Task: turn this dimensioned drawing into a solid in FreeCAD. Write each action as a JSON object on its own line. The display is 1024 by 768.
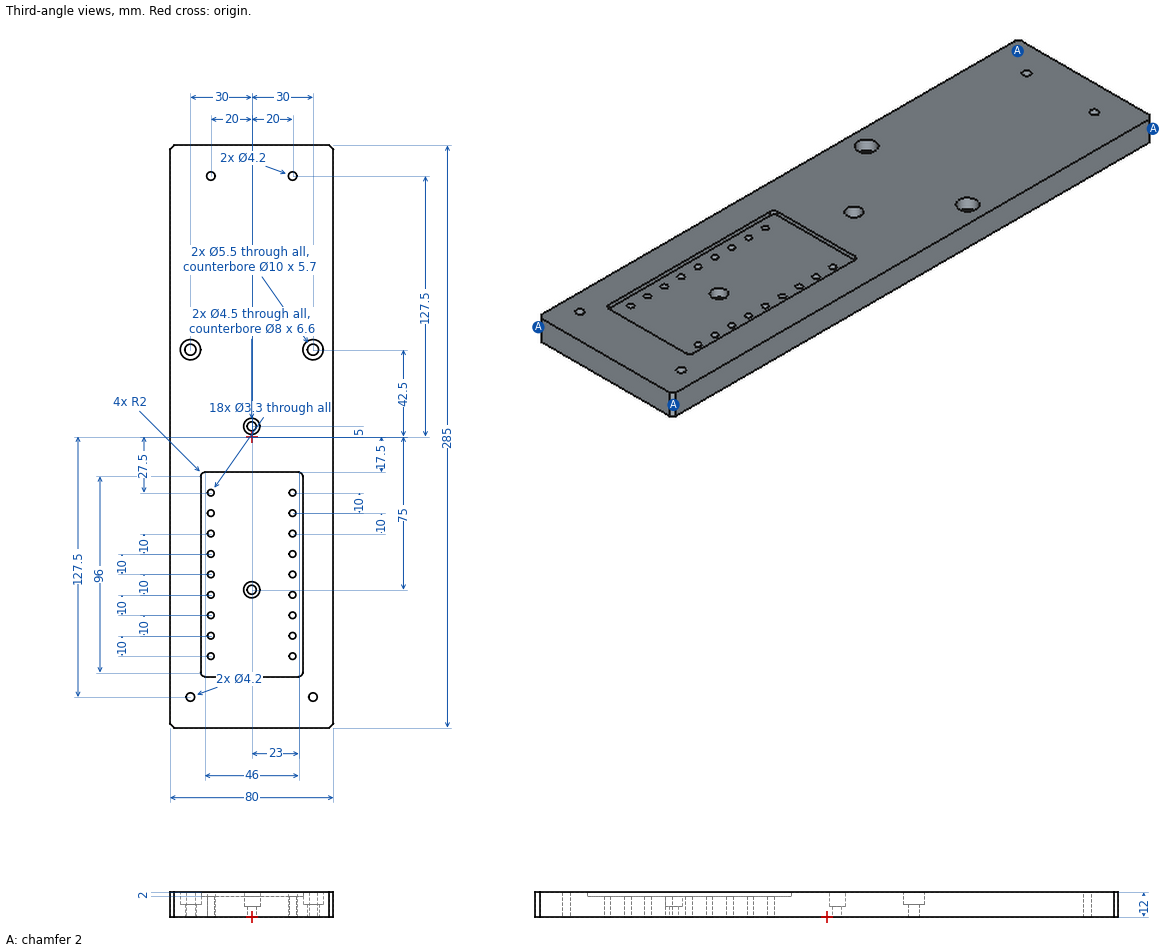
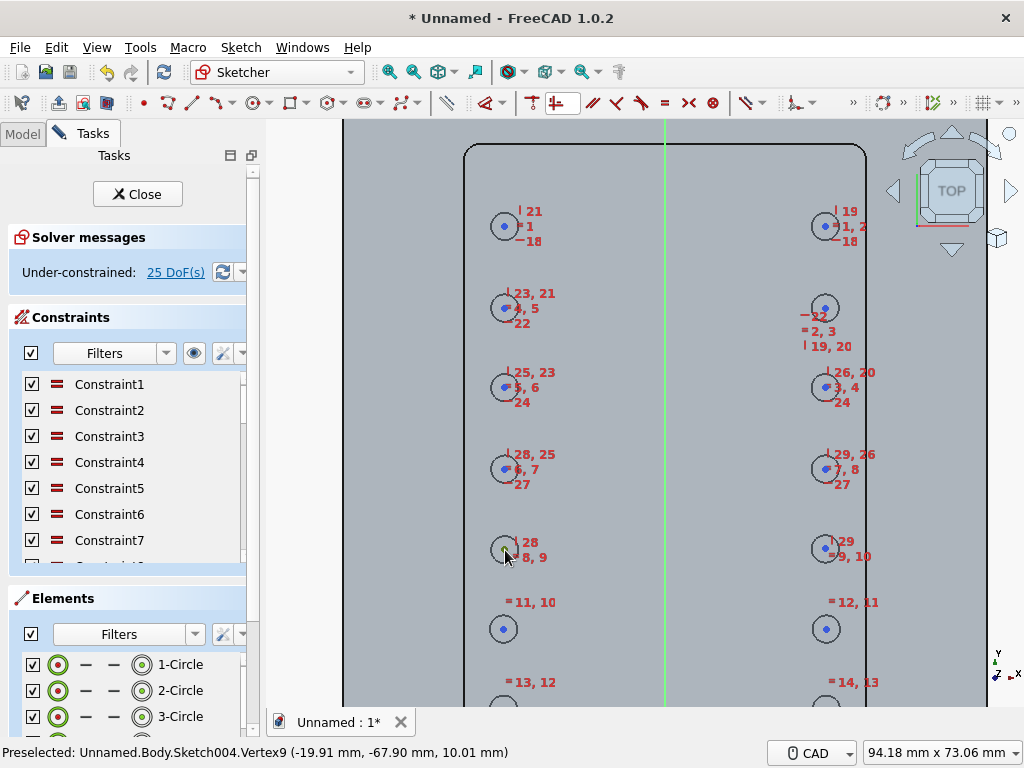
{"action": "left_click", "coordinate": [825, 549]}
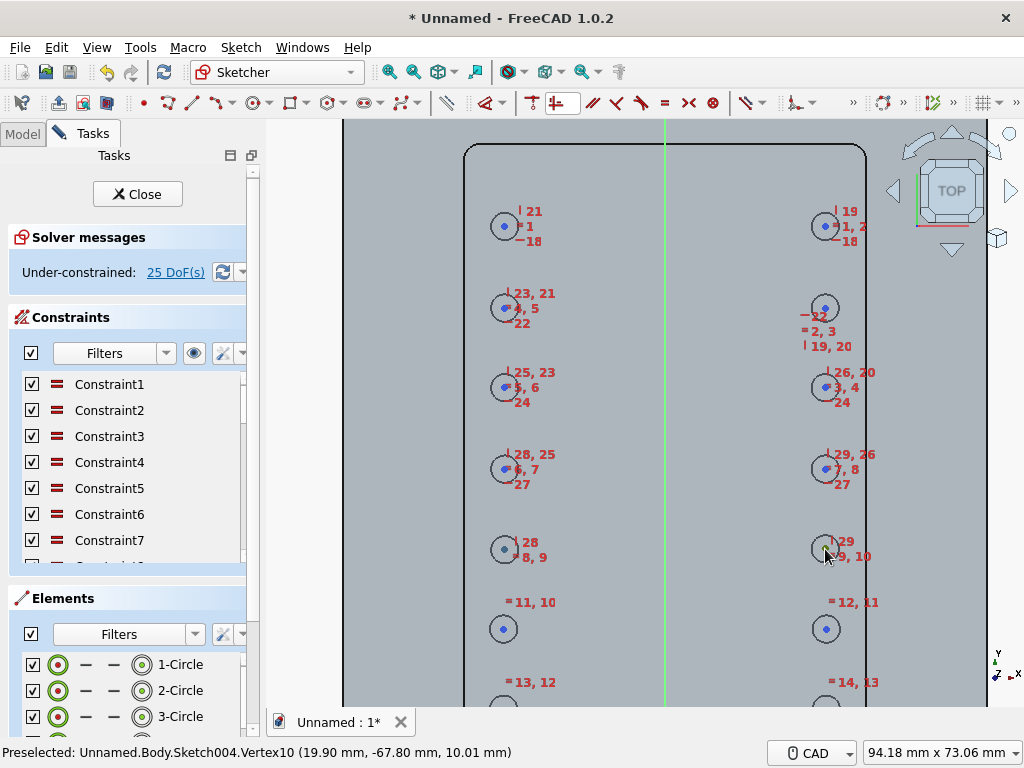
{"action": "key", "text": "h"}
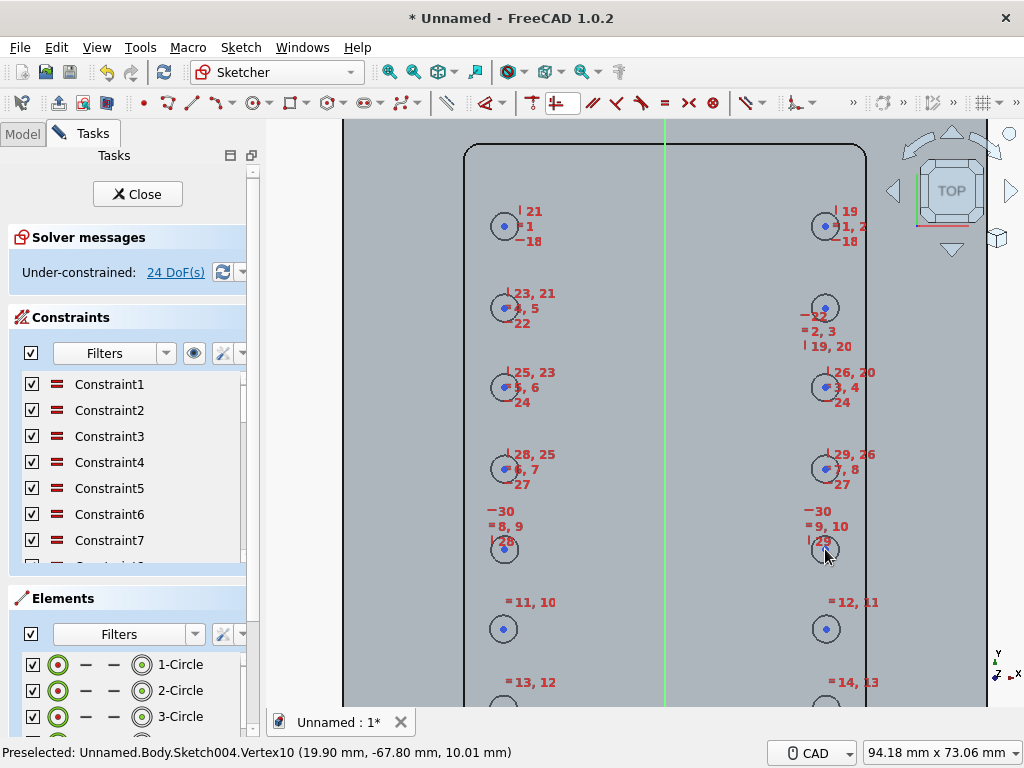
{"action": "left_click", "coordinate": [505, 550]}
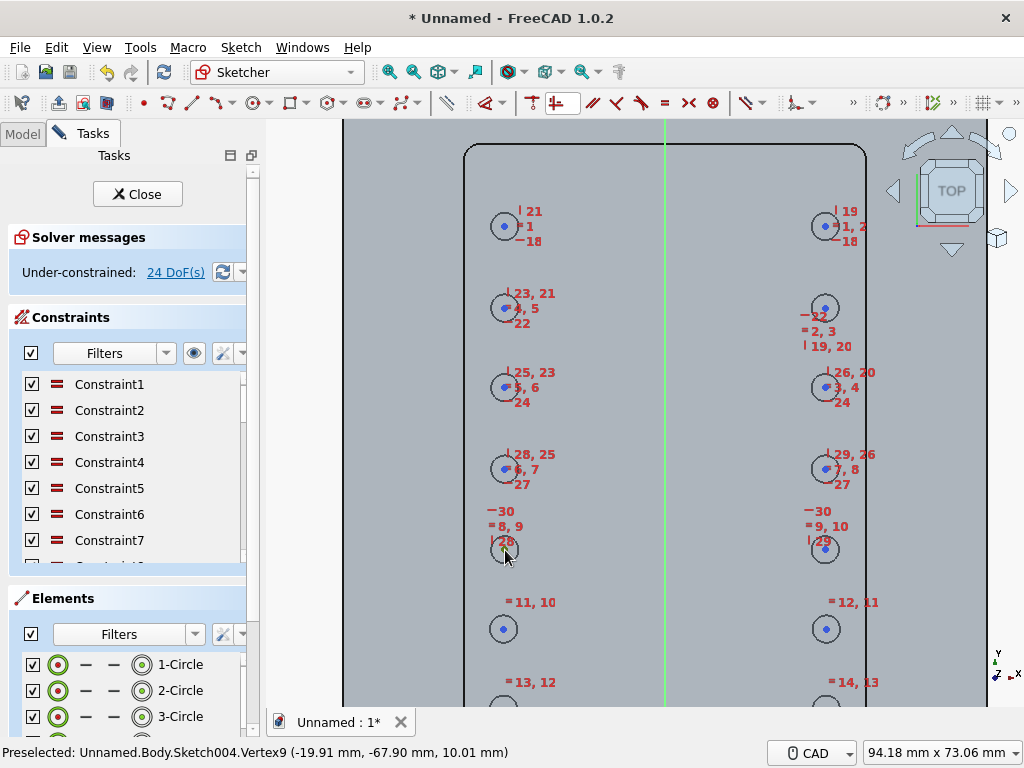
{"action": "left_click", "coordinate": [504, 629]}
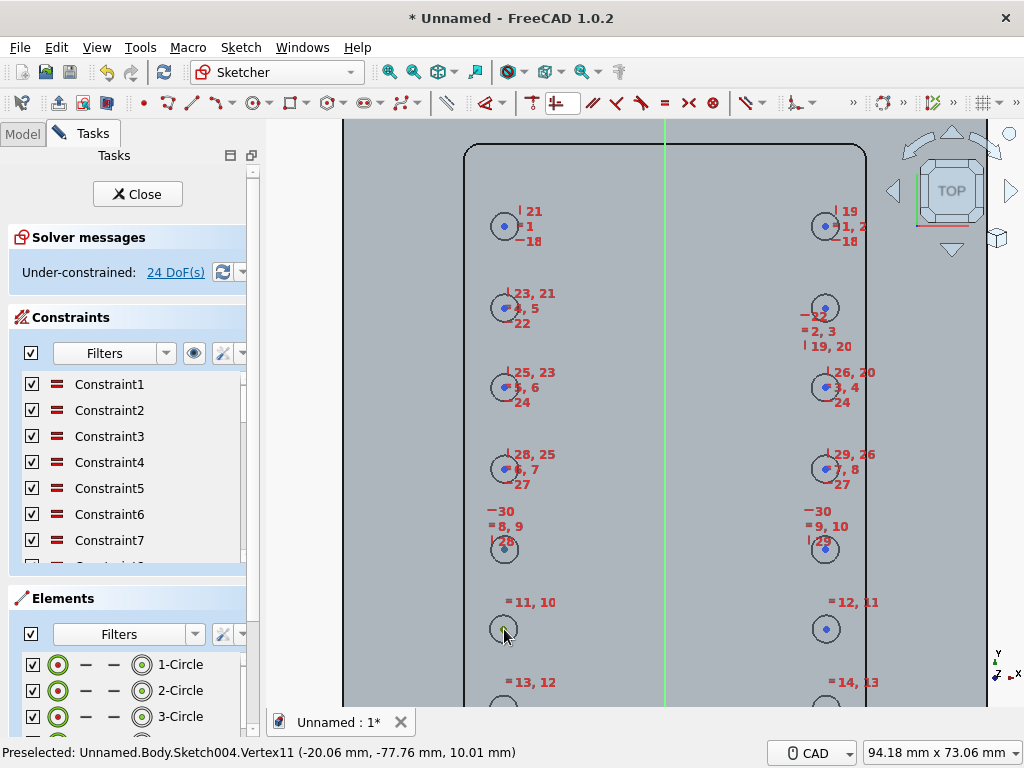
{"action": "left_click", "coordinate": [574, 104]}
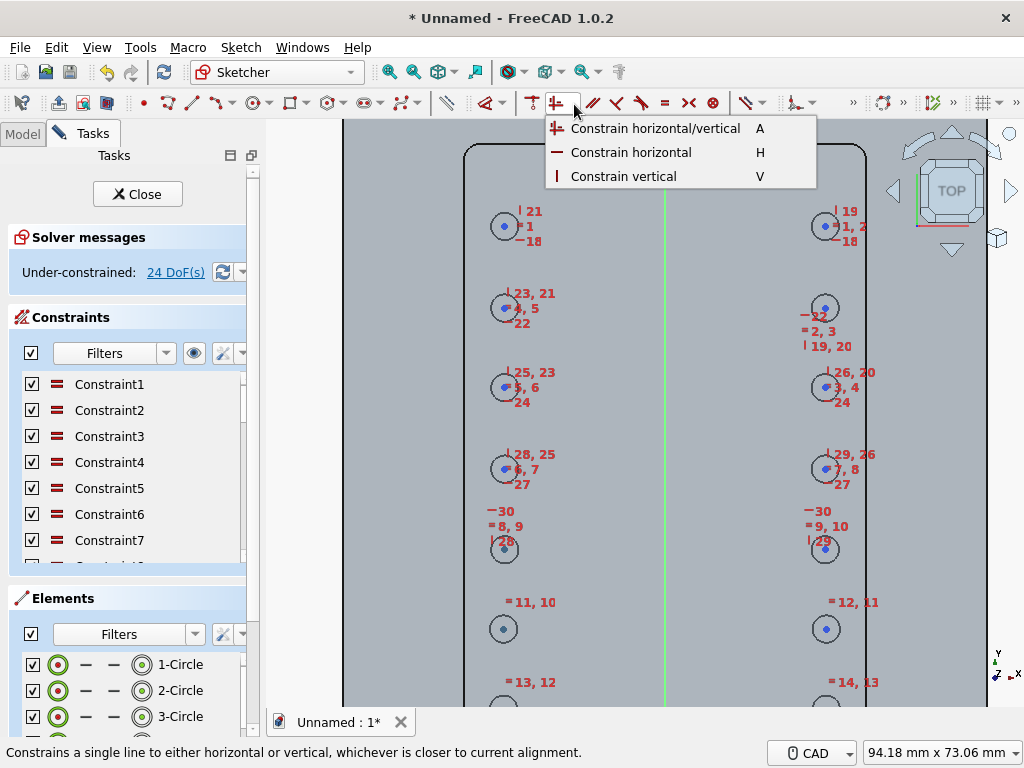
{"action": "left_click", "coordinate": [681, 176]}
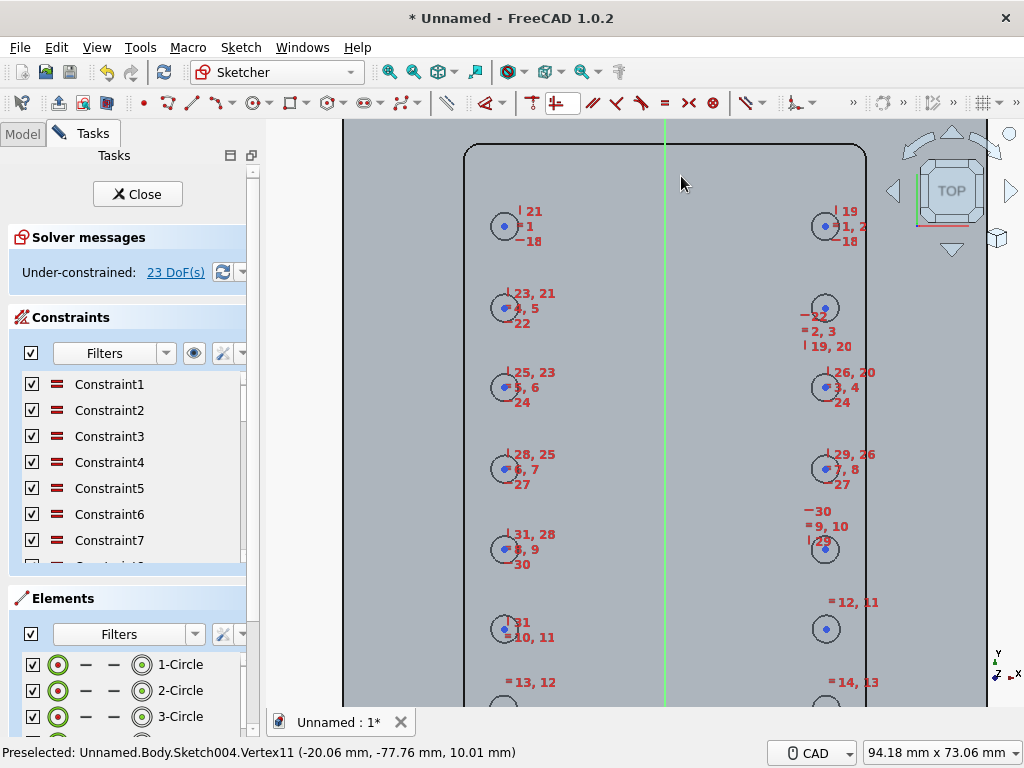
{"action": "left_click", "coordinate": [825, 550]}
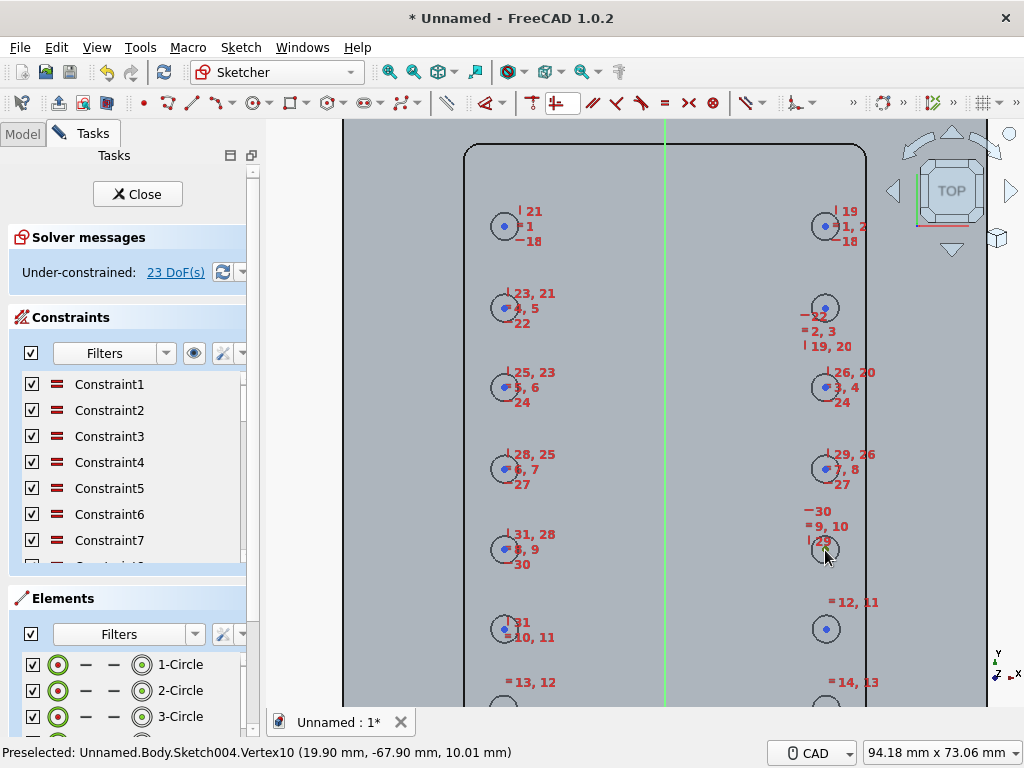
{"action": "left_click", "coordinate": [826, 629]}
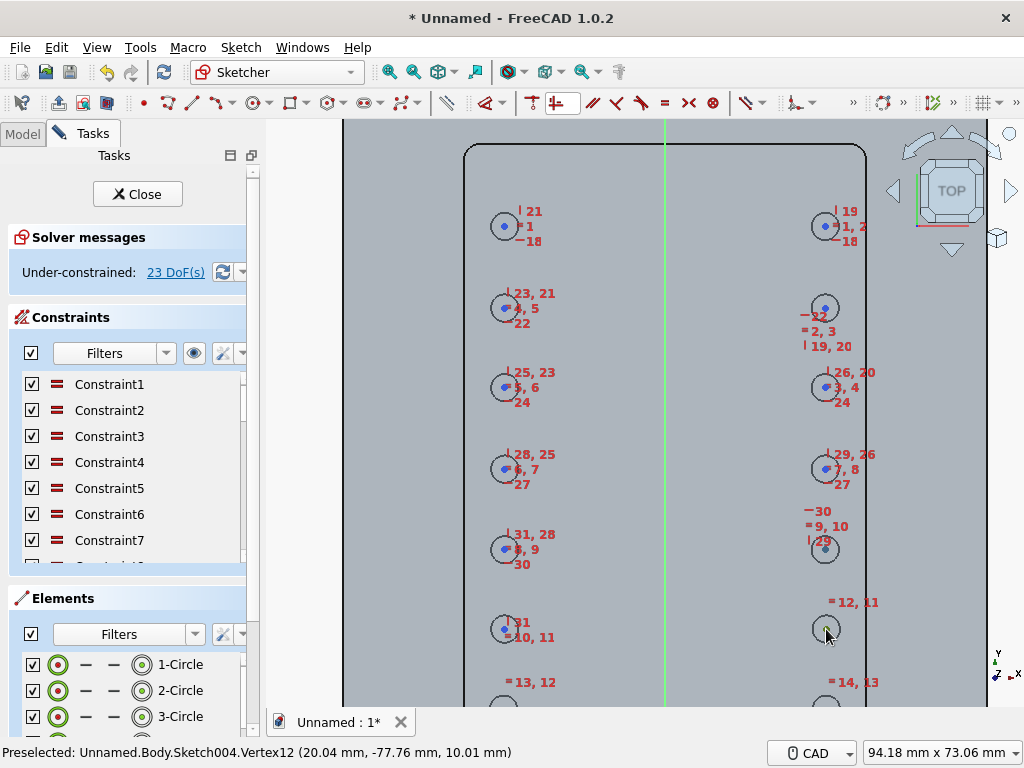
{"action": "key", "text": "v"}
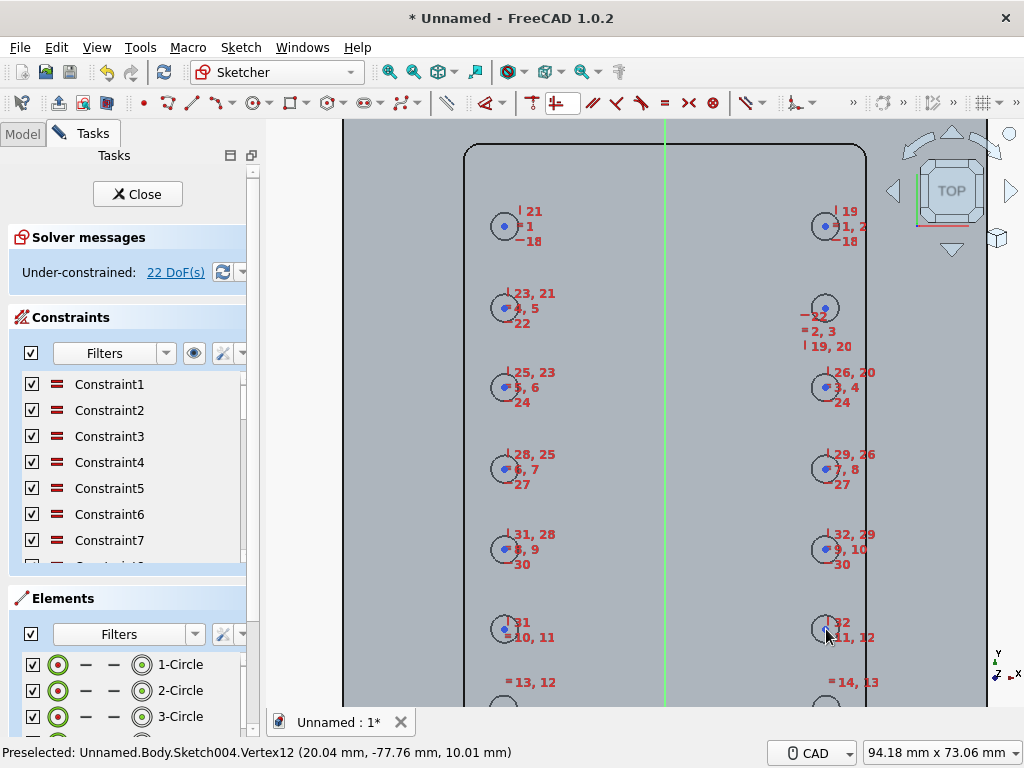
{"action": "scroll", "coordinate": [505, 629], "scroll_direction": "up", "scroll_amount": 4}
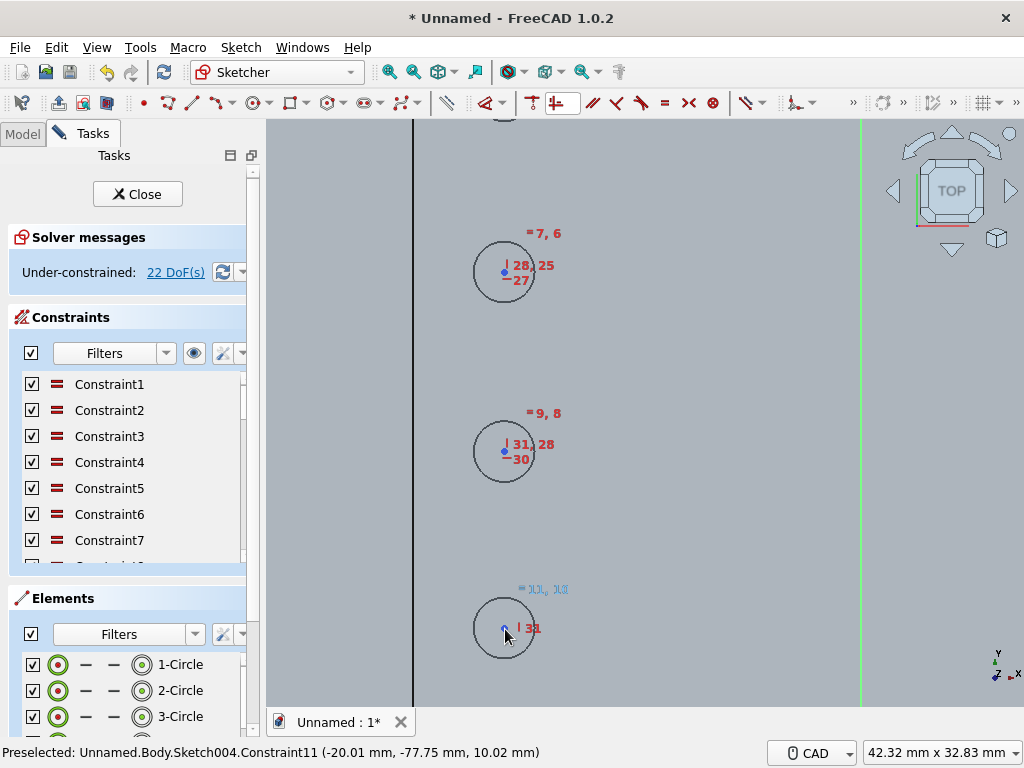
{"action": "left_click", "coordinate": [504, 628]}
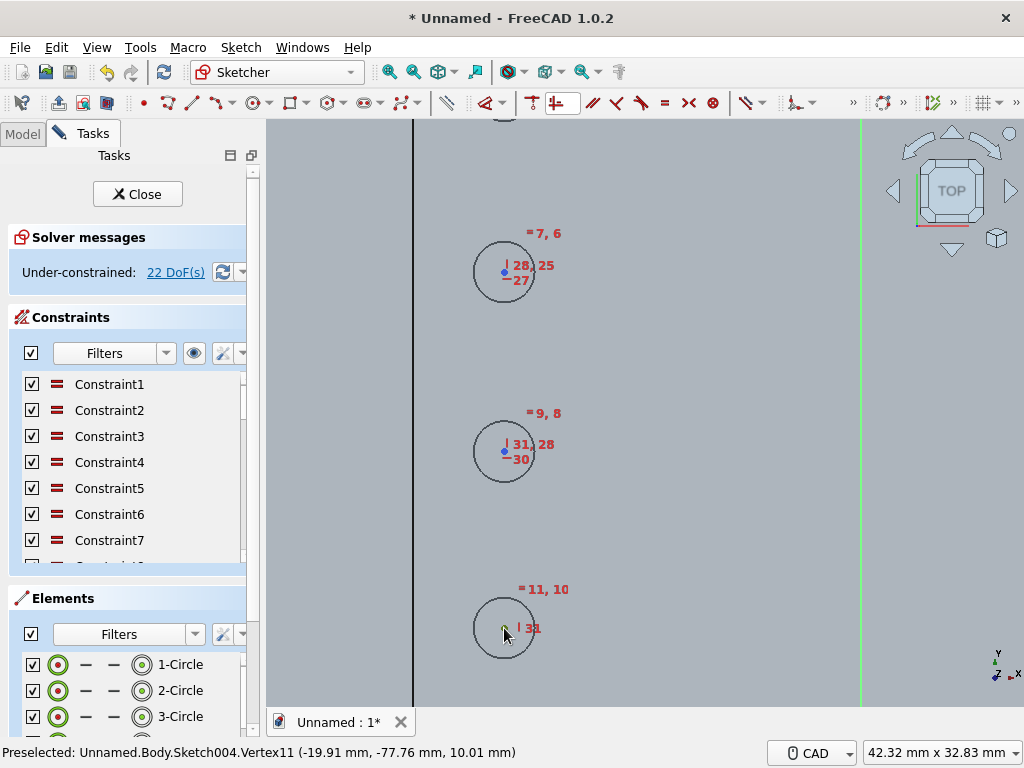
{"action": "scroll", "coordinate": [505, 464], "scroll_direction": "down", "scroll_amount": 8}